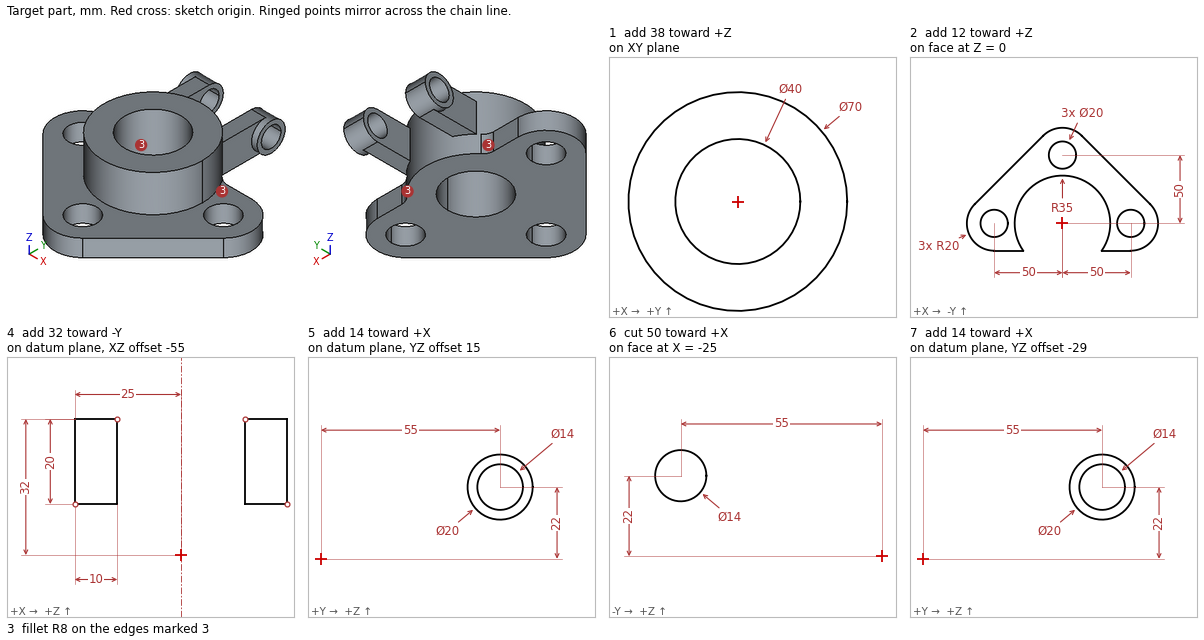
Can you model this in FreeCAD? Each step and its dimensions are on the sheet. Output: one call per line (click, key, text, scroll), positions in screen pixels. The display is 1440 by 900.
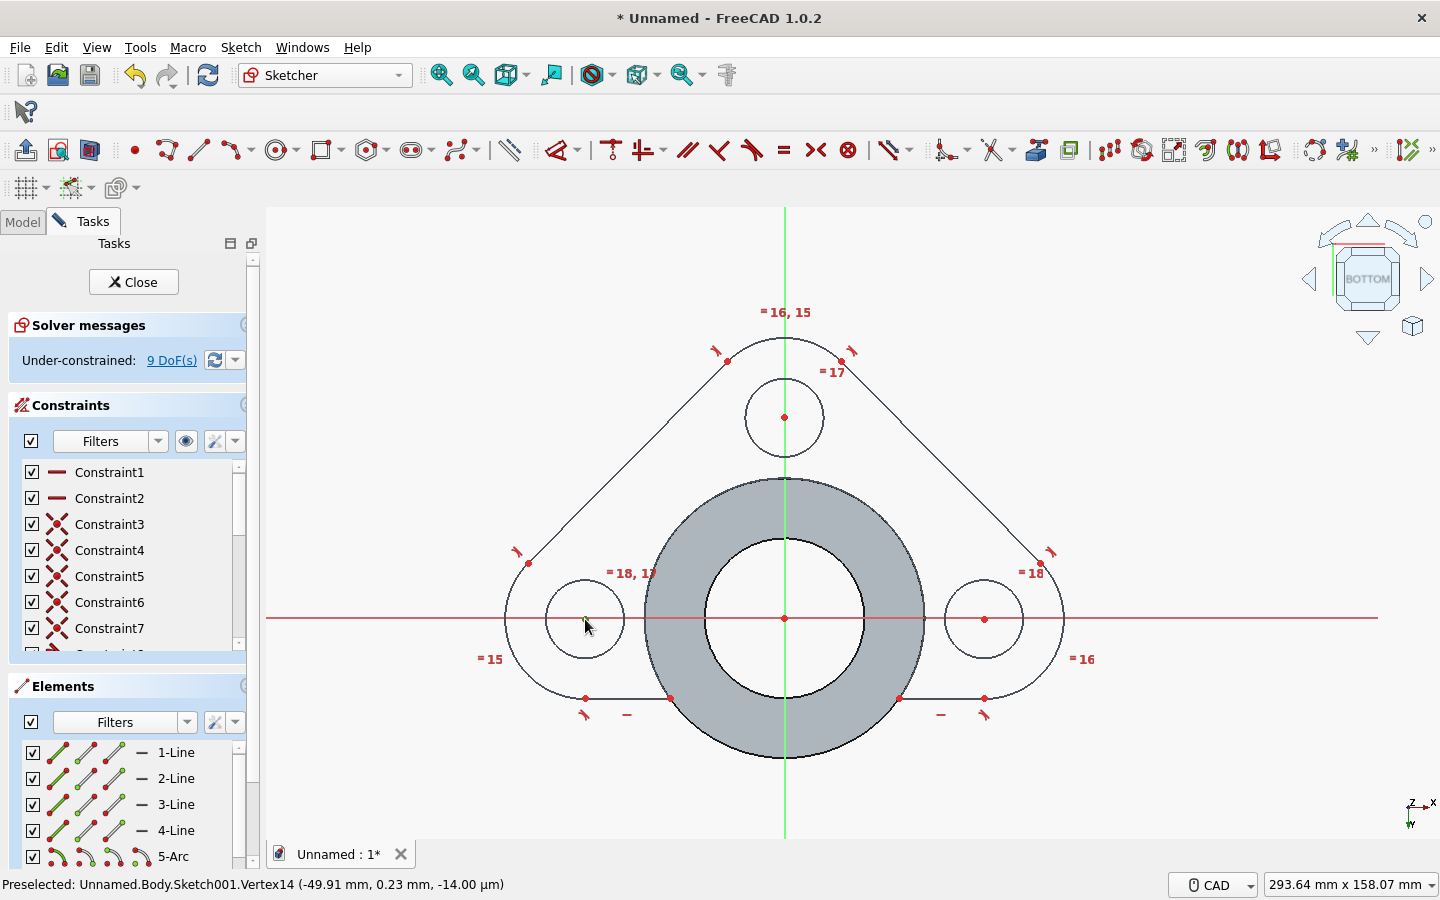
click(364, 618)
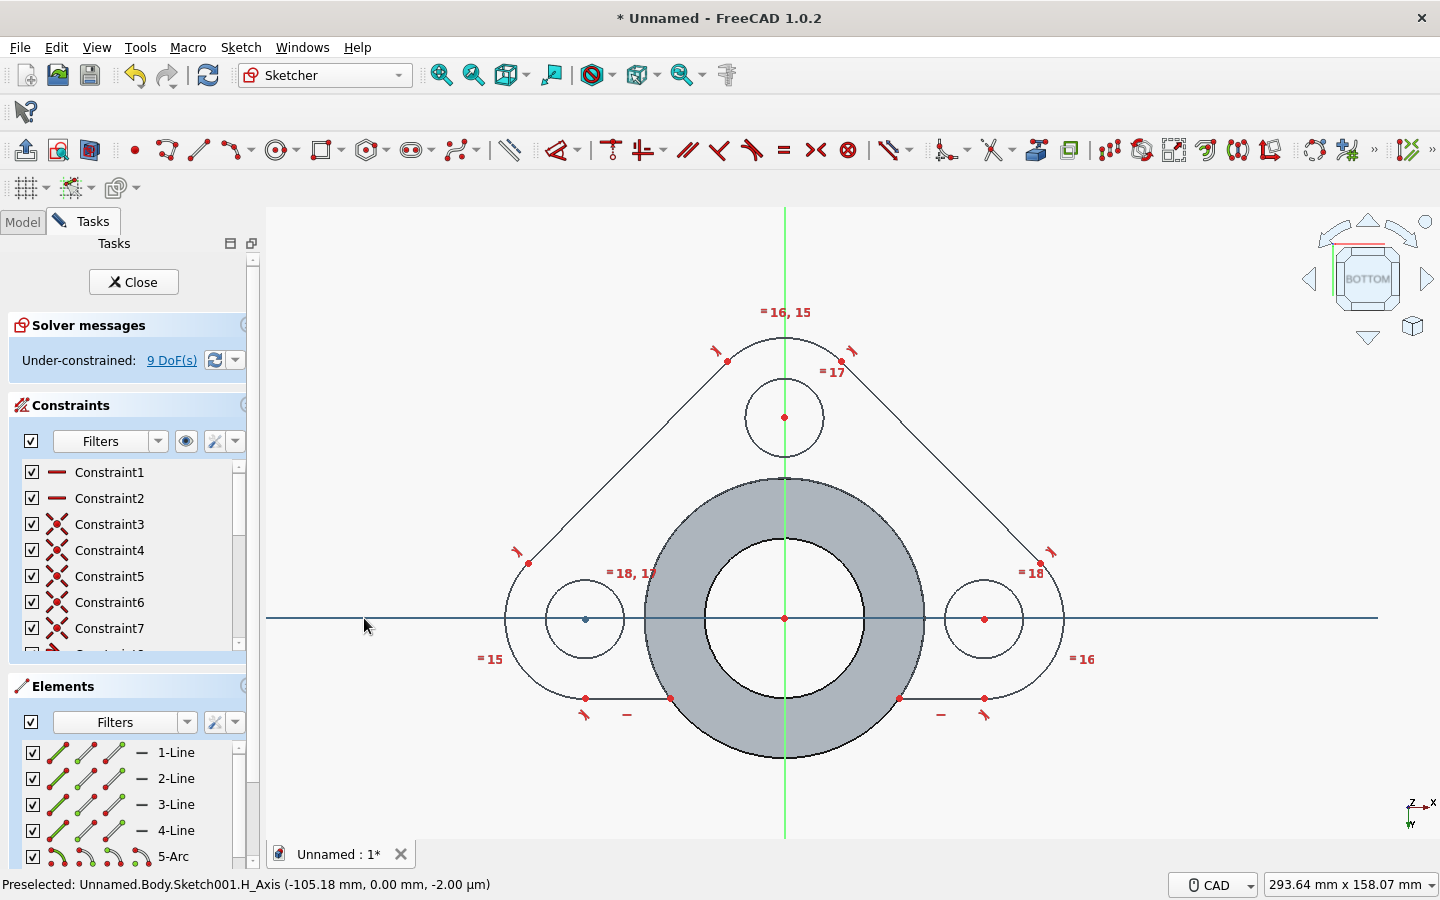
key(c)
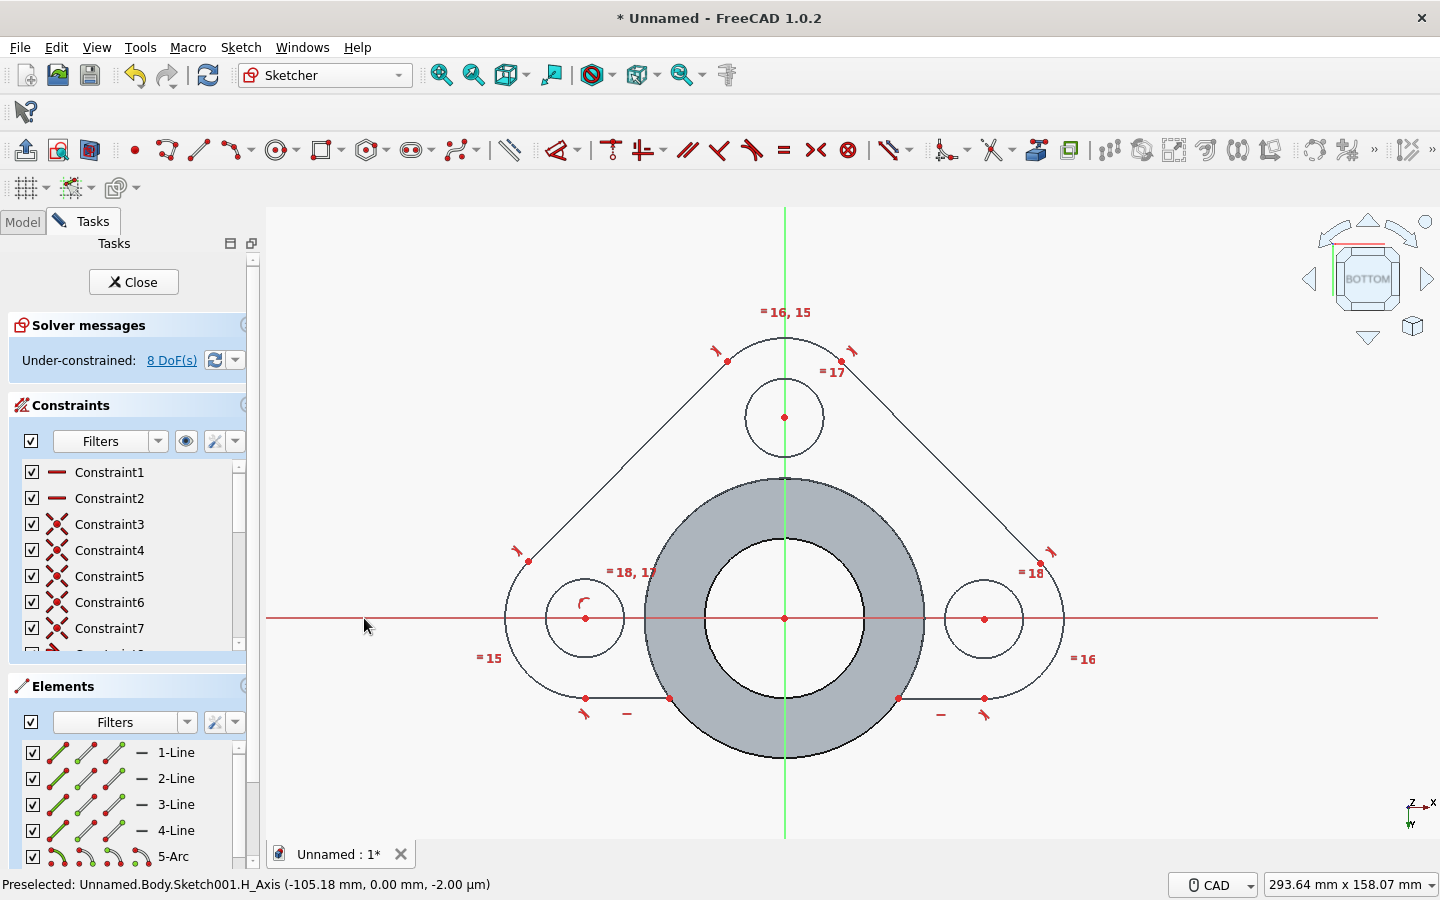
click(785, 418)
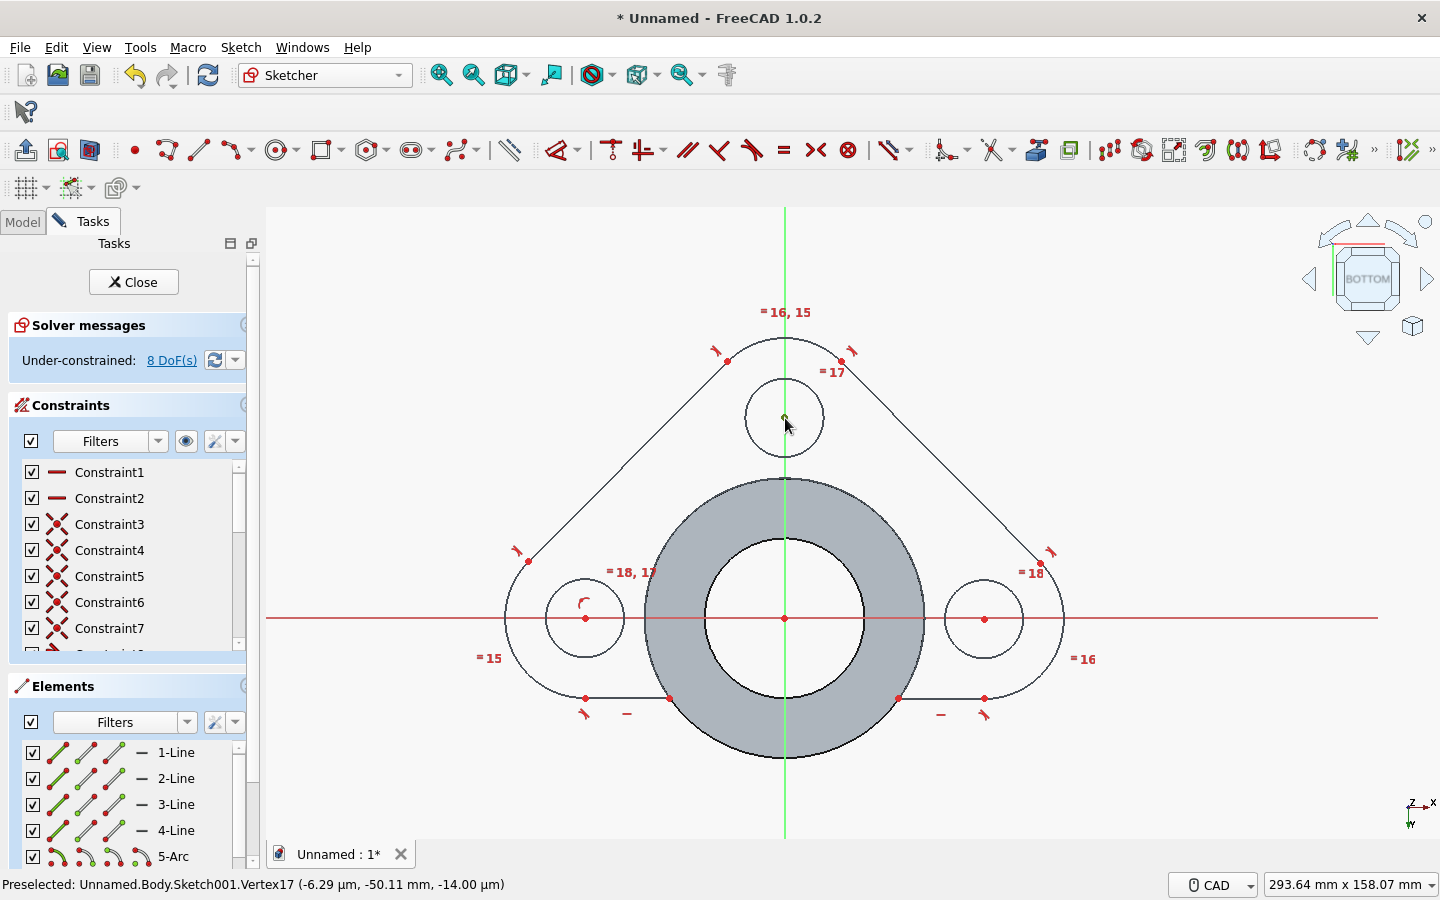
click(785, 770)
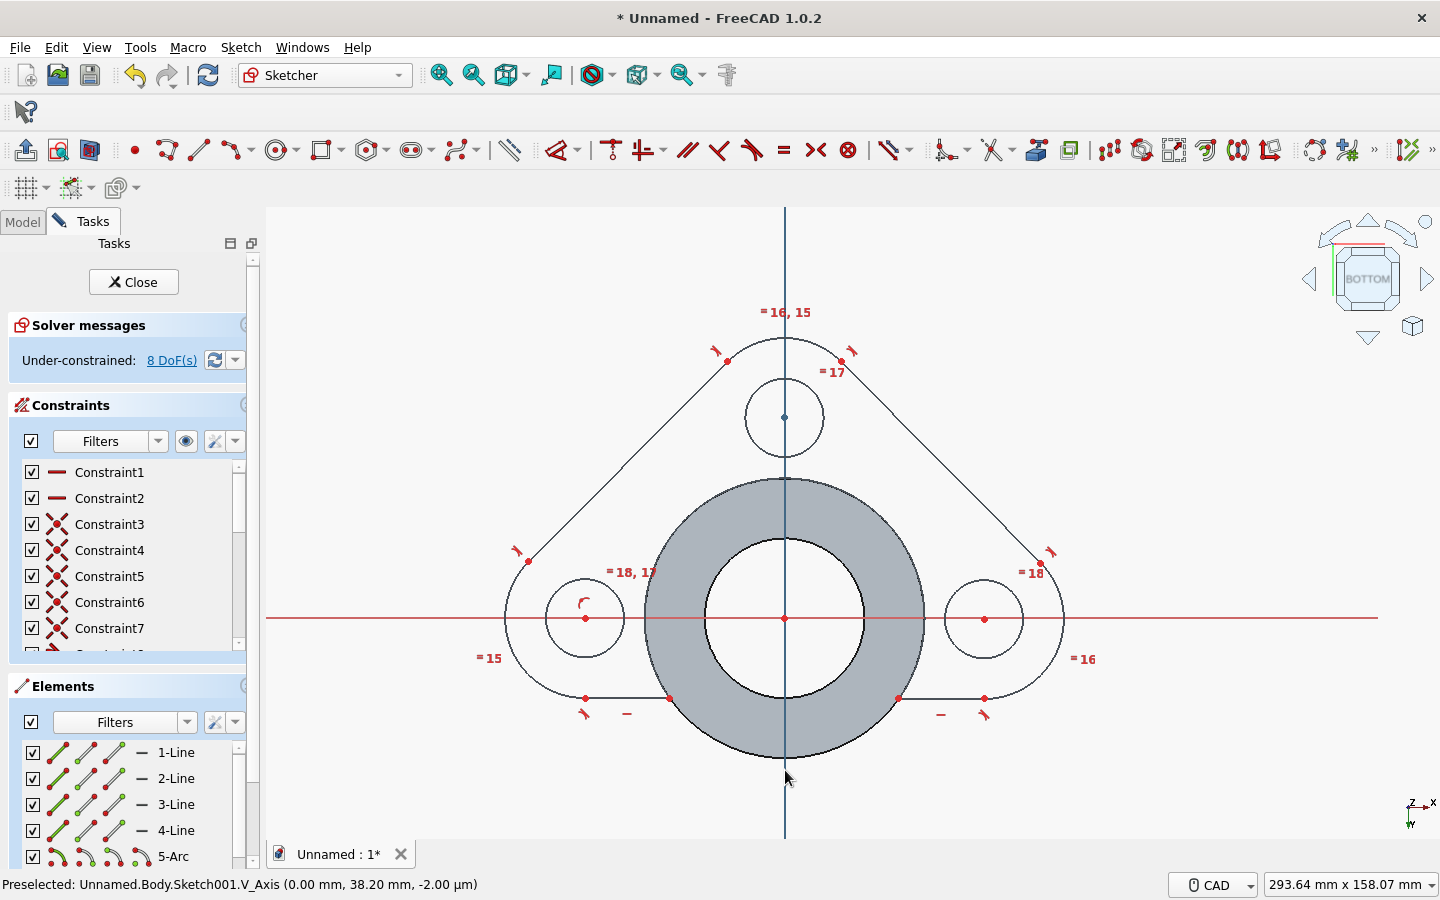
key(c)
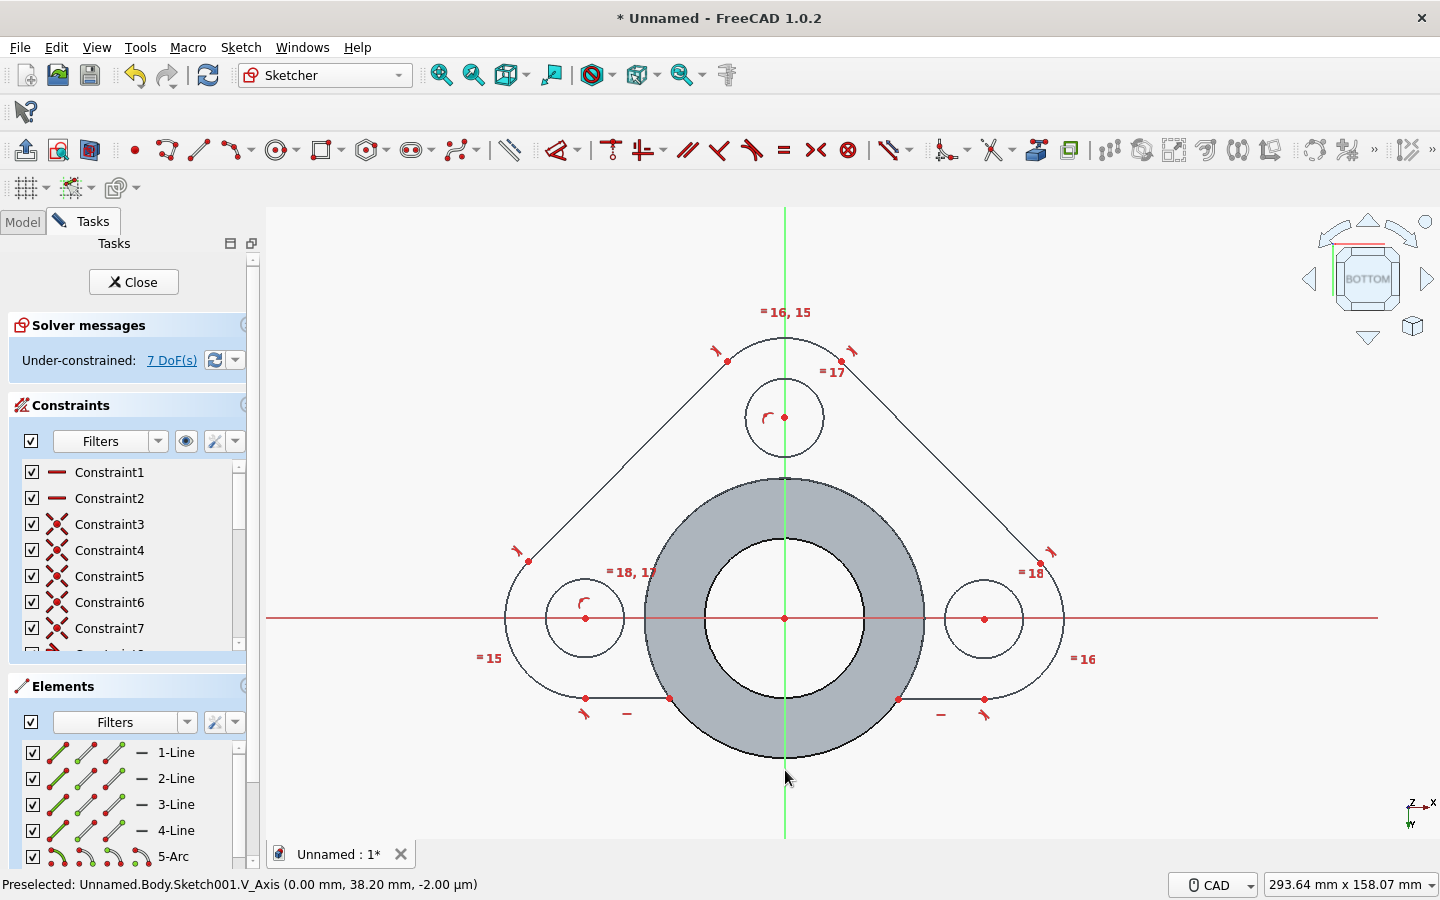
click(984, 619)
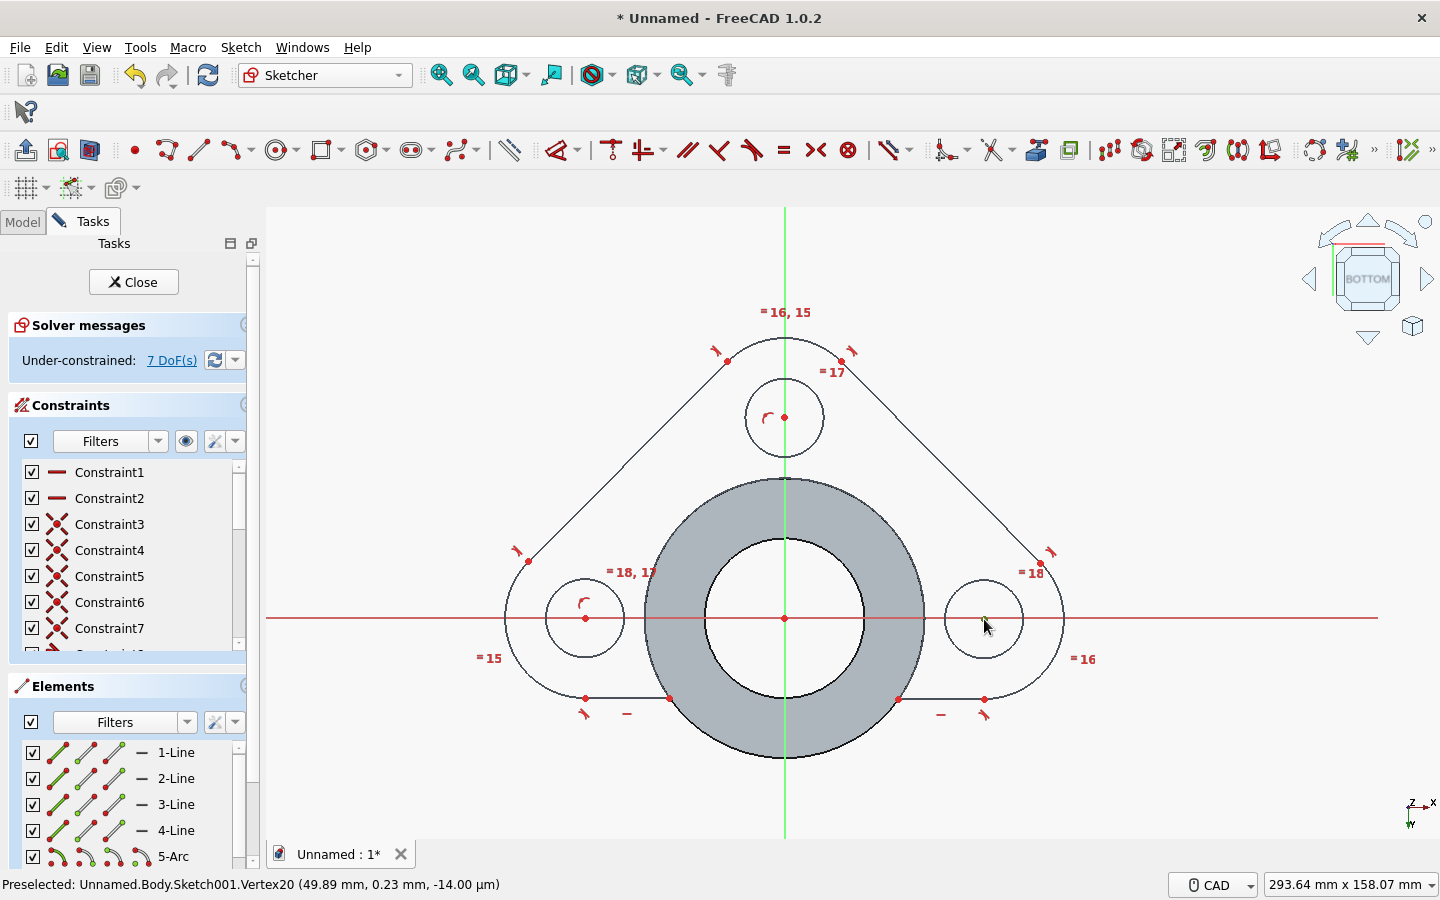
click(364, 618)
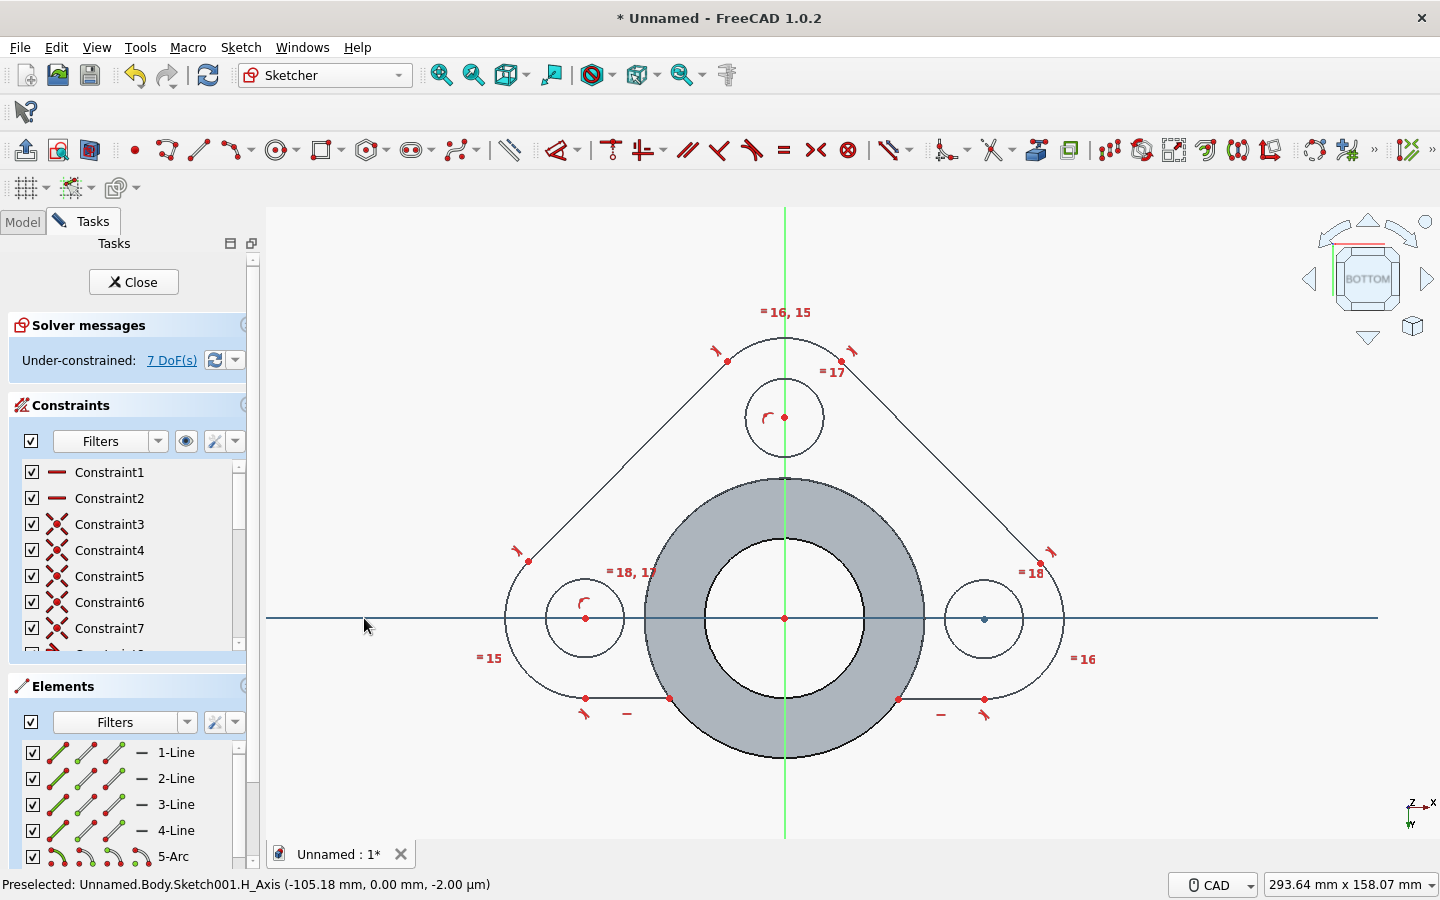
key(c)